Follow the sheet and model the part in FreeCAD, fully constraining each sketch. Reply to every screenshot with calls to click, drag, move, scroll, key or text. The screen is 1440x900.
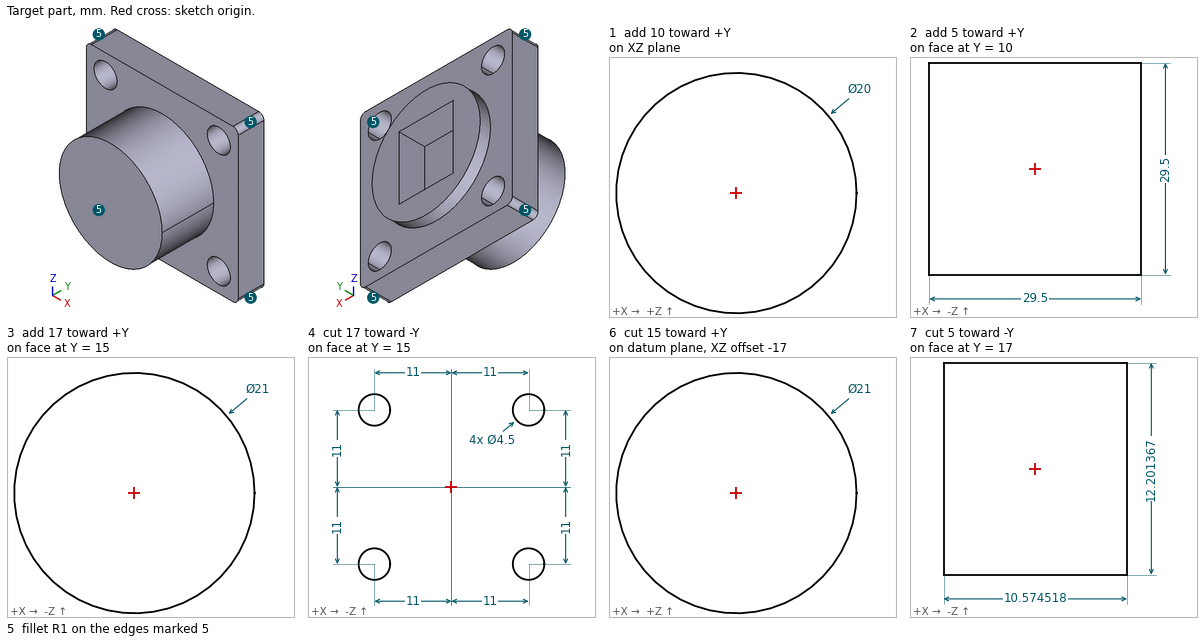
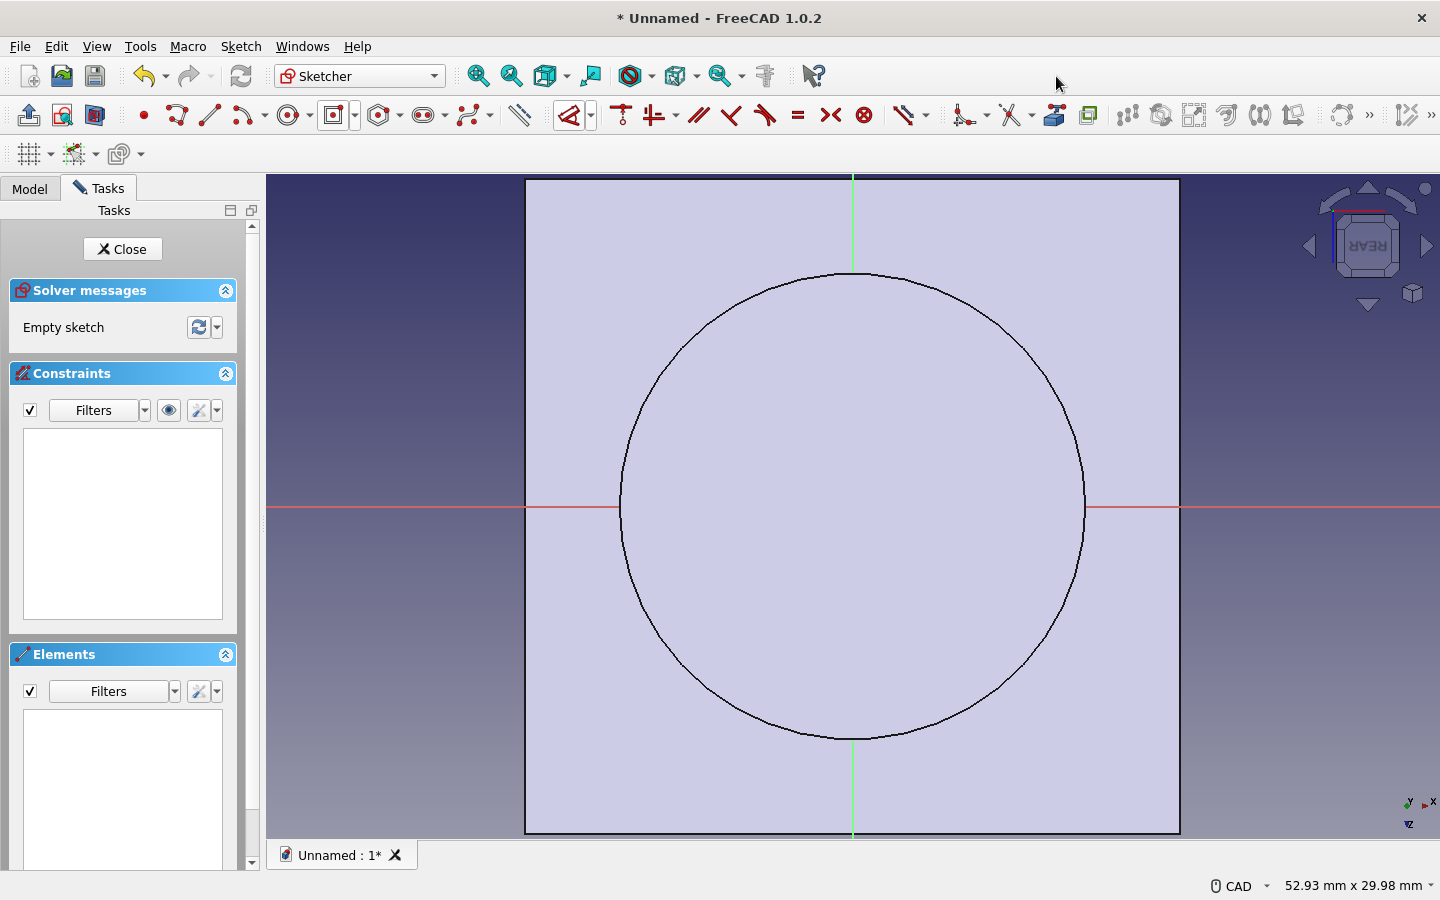
click(95, 116)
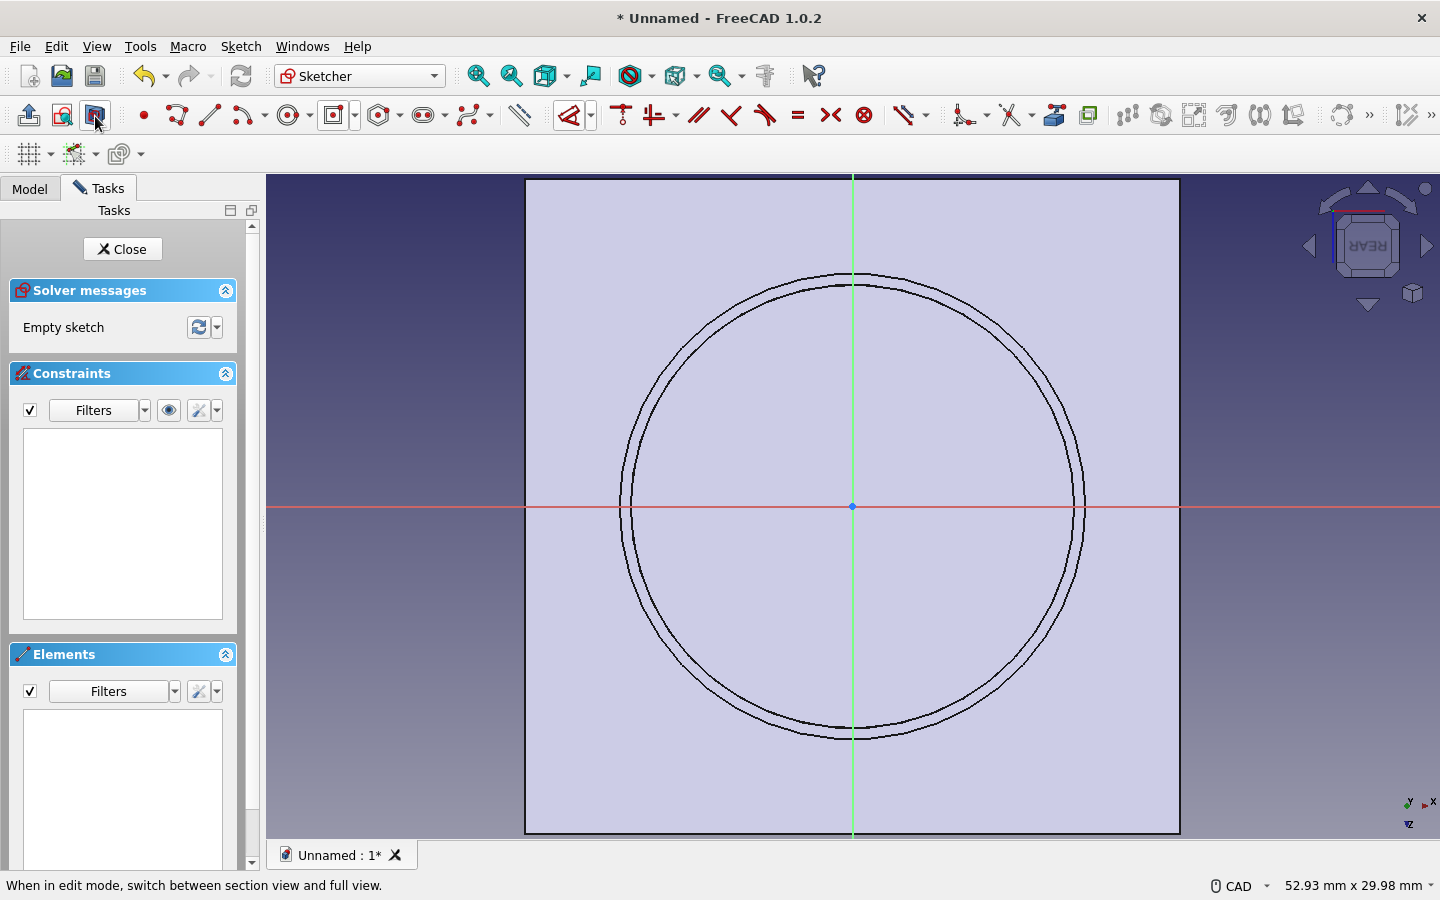
scroll(646, 507, down, 2)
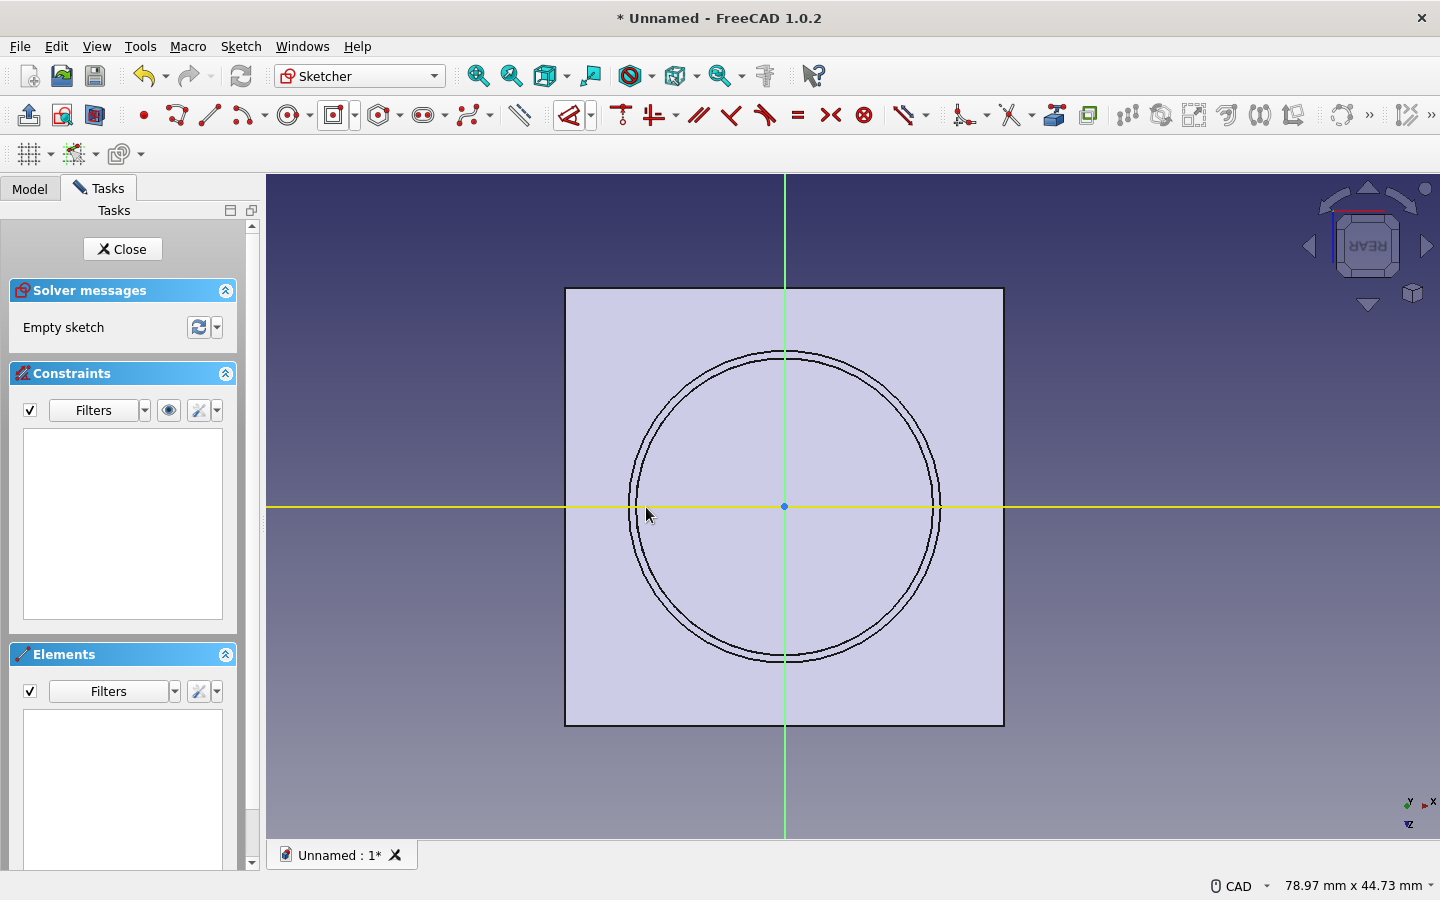
click(288, 116)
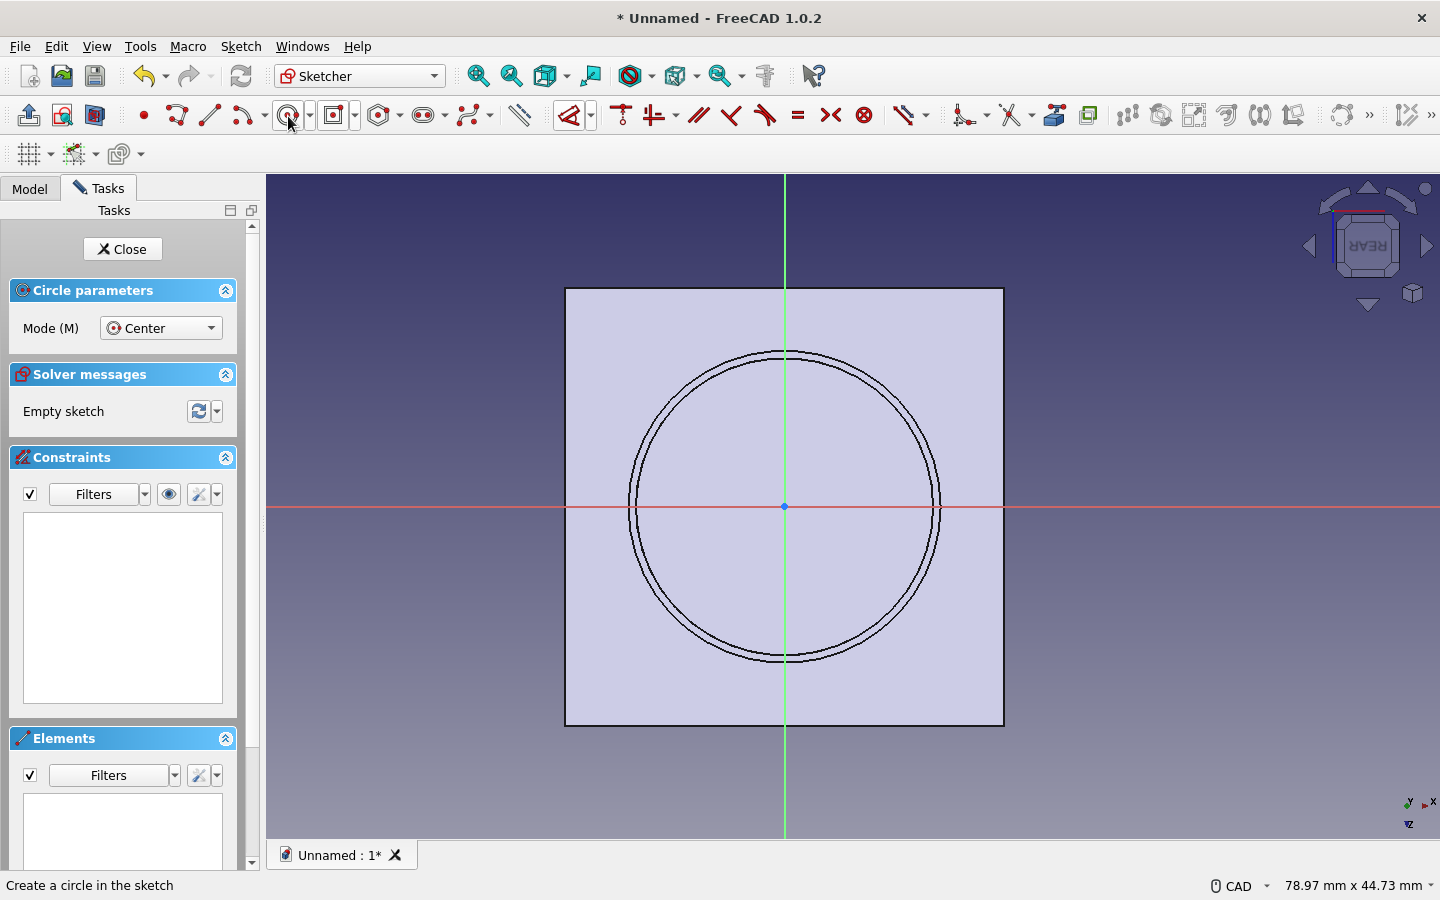
click(948, 343)
click(972, 320)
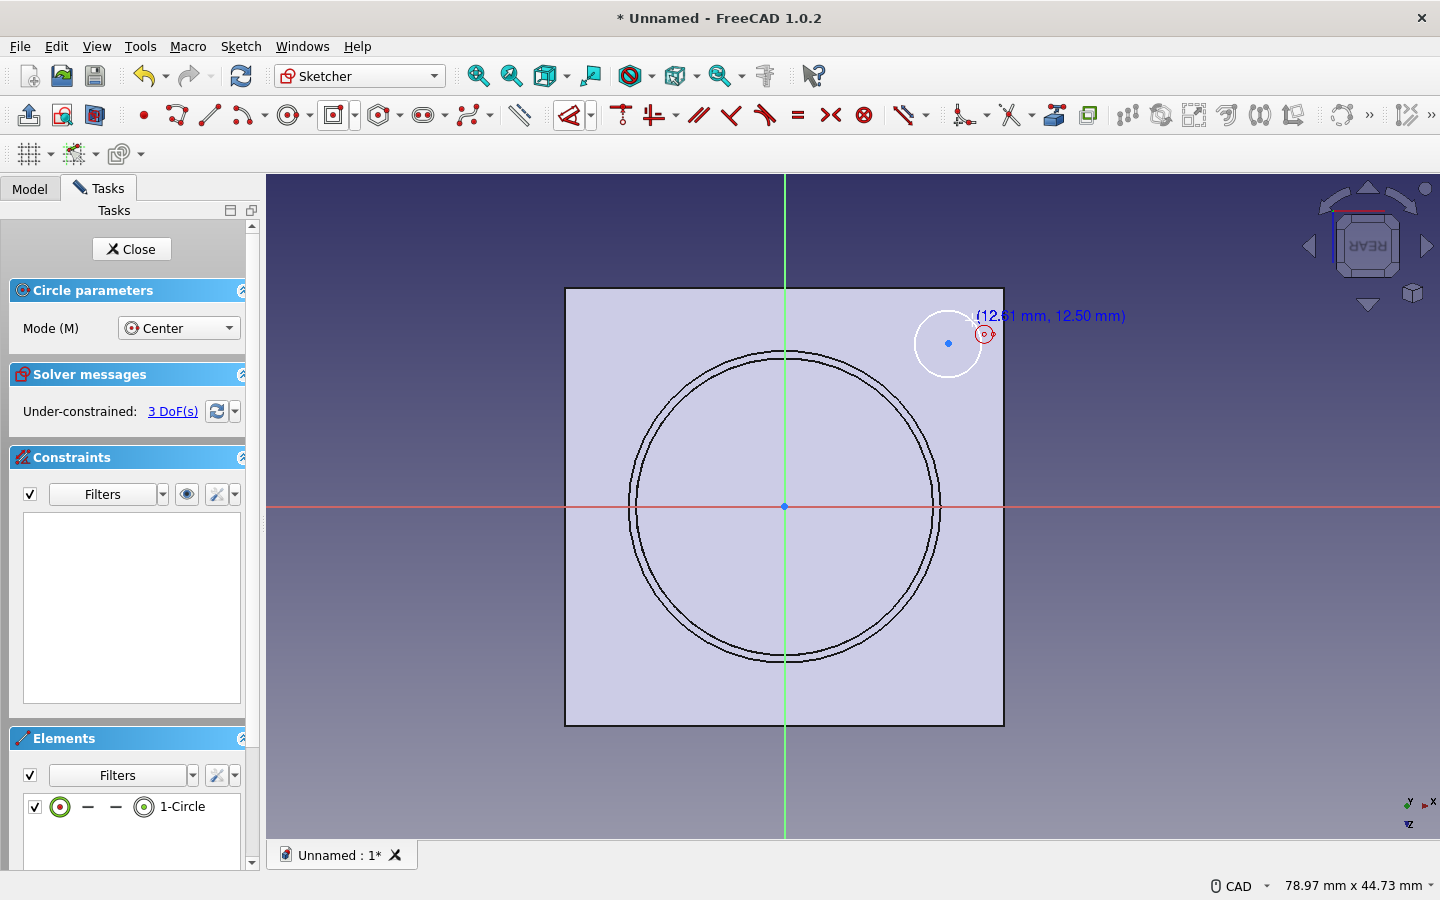
click(621, 343)
click(645, 320)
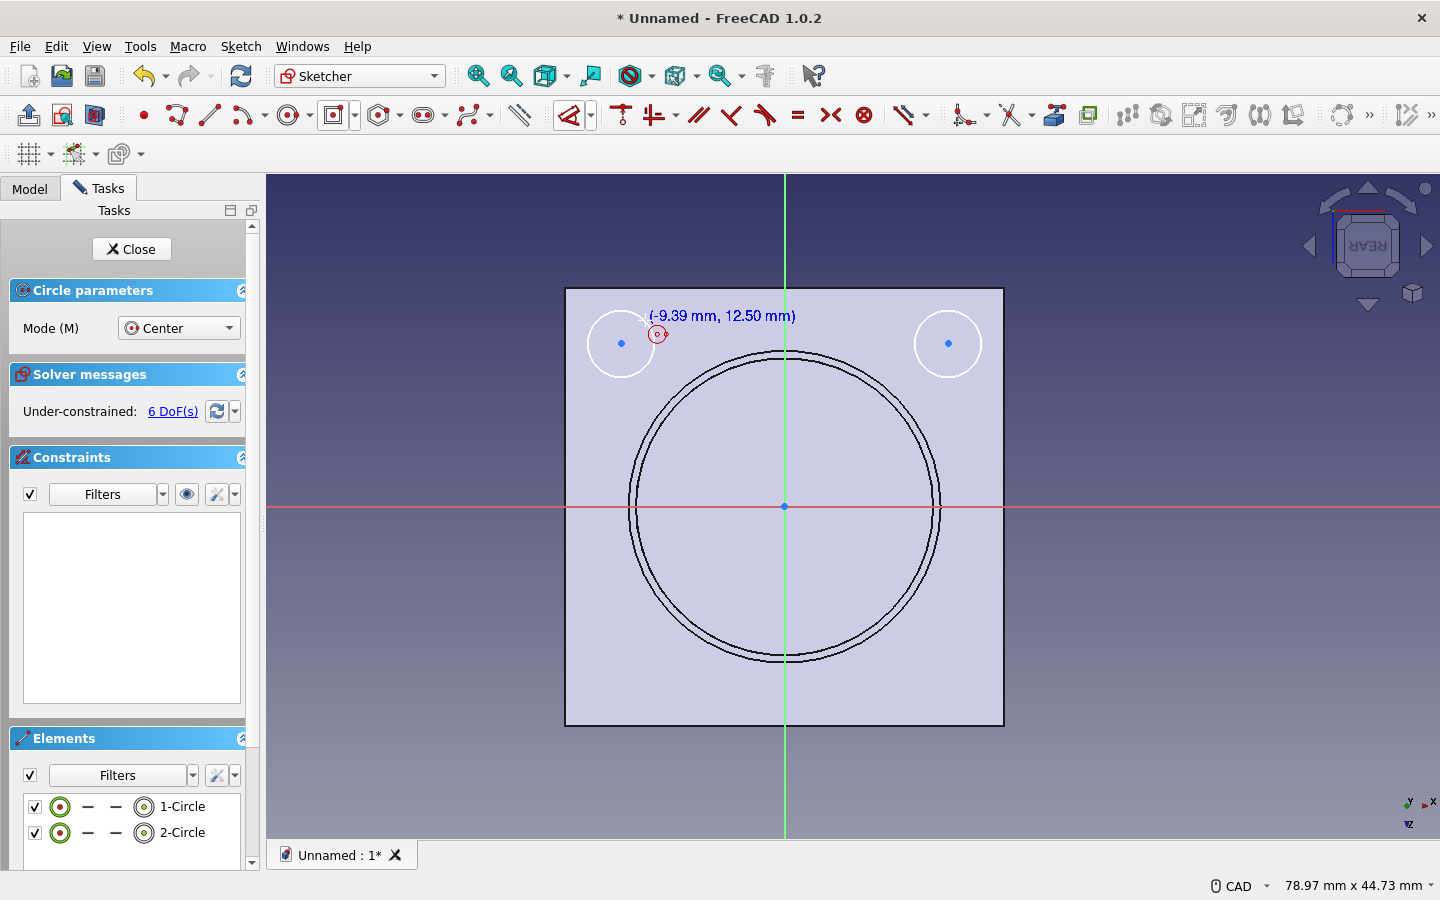
click(621, 670)
click(645, 647)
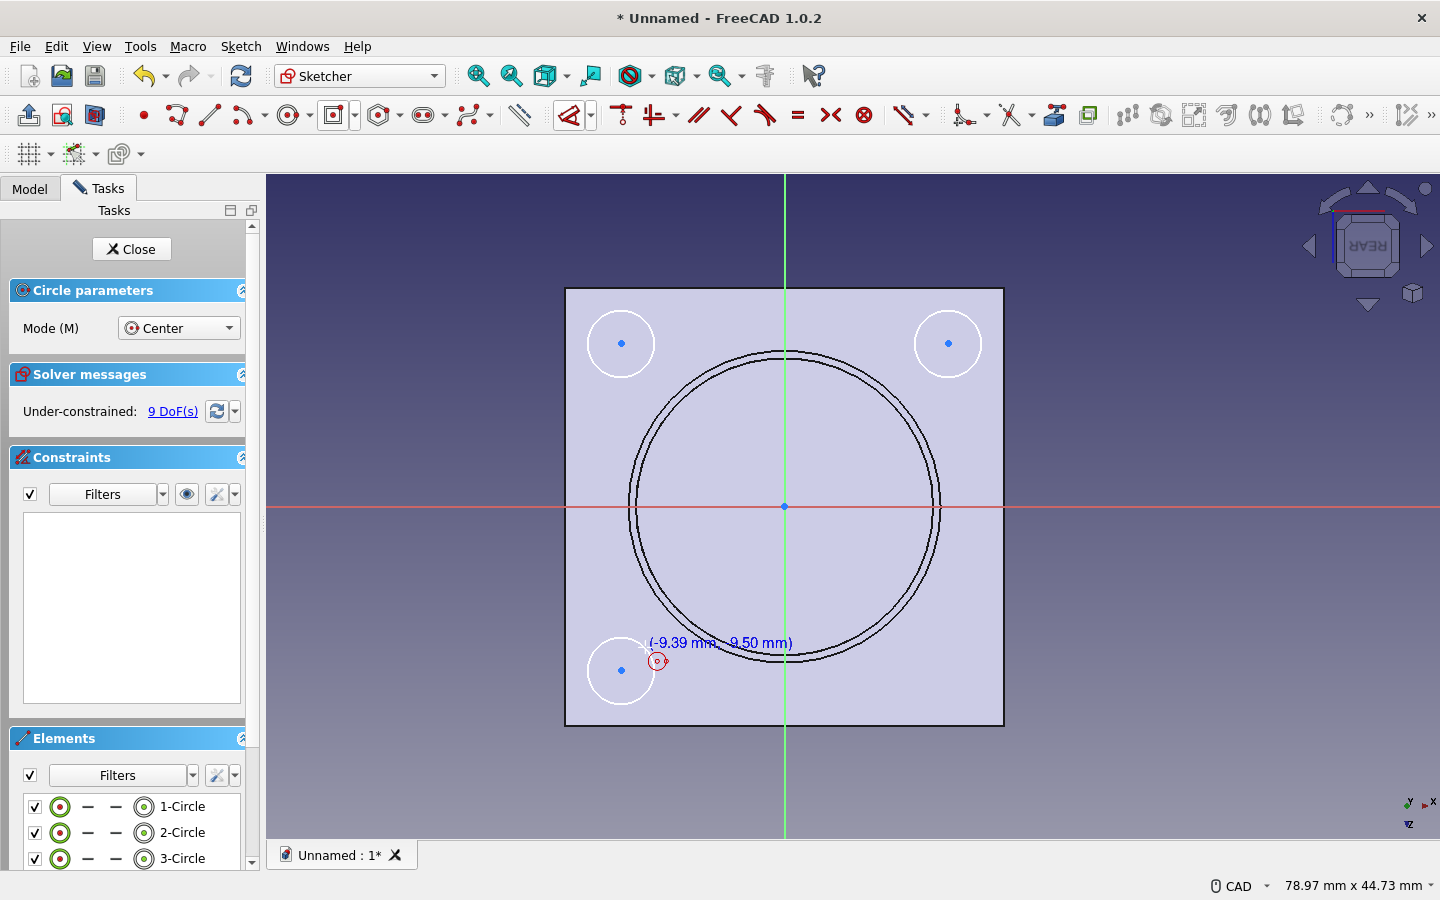
click(948, 670)
click(972, 647)
key(Escape)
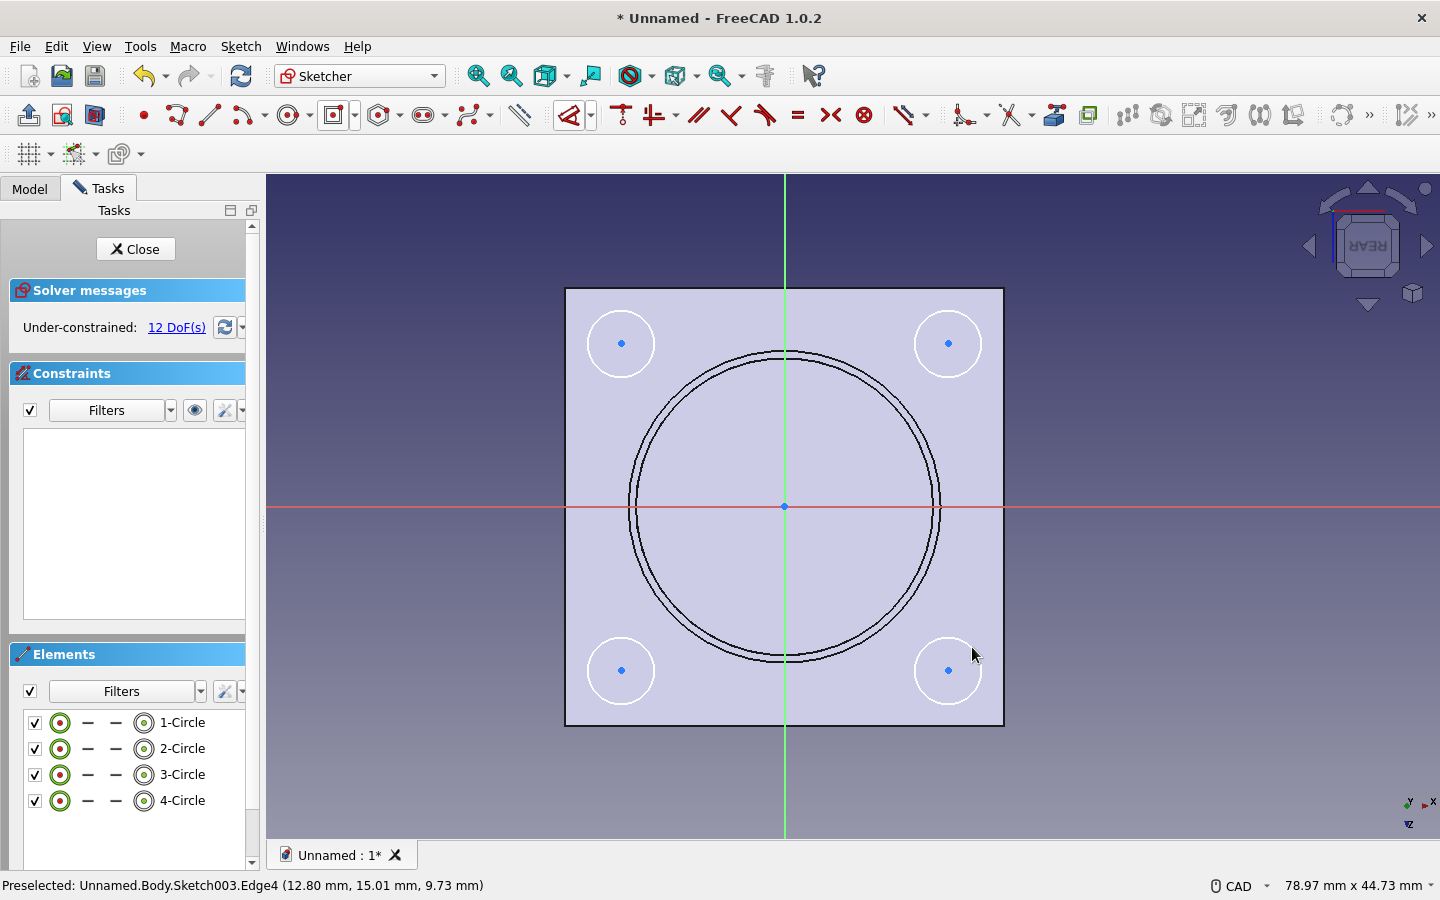
click(971, 320)